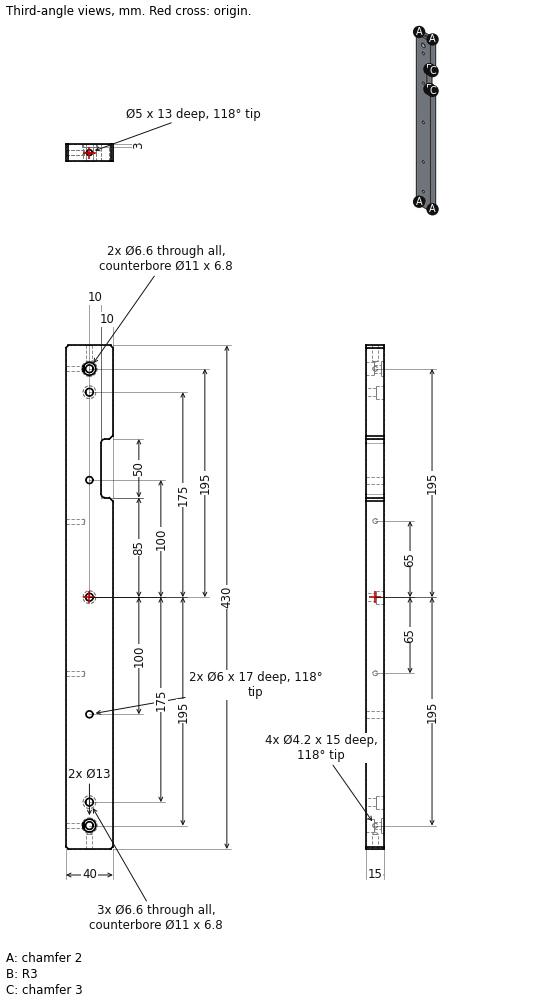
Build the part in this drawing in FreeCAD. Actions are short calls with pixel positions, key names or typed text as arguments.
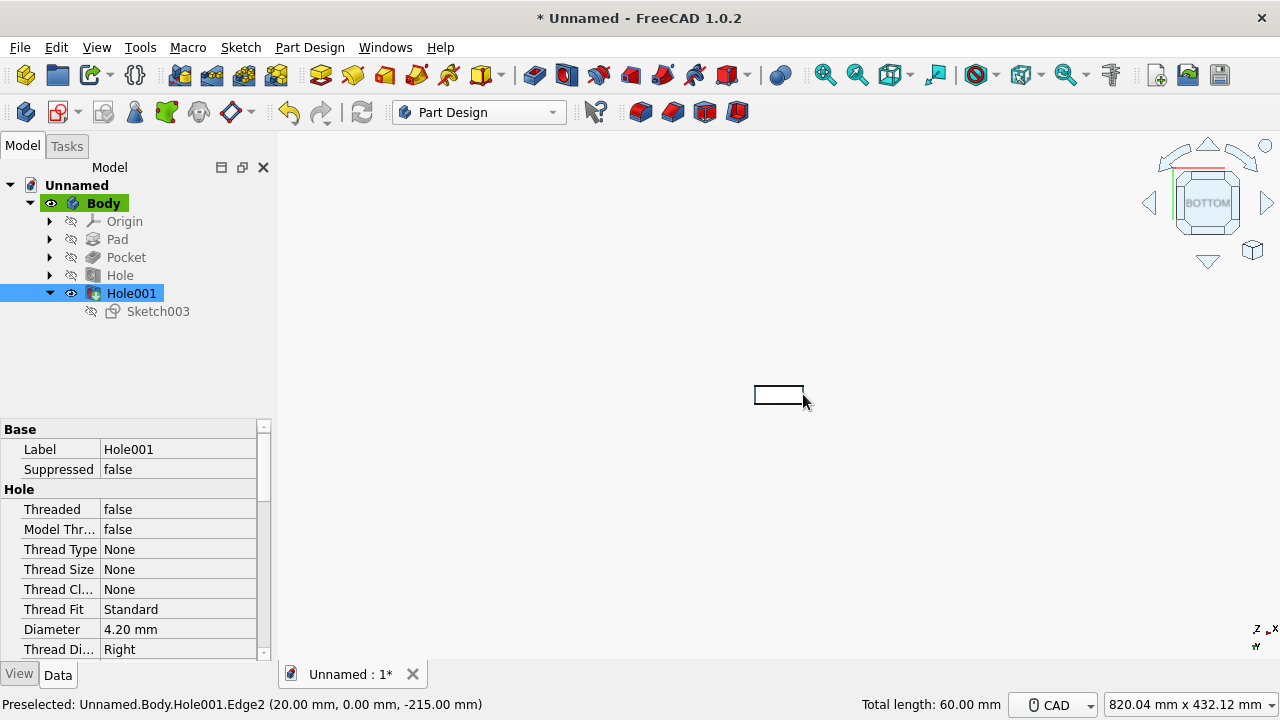
click(674, 112)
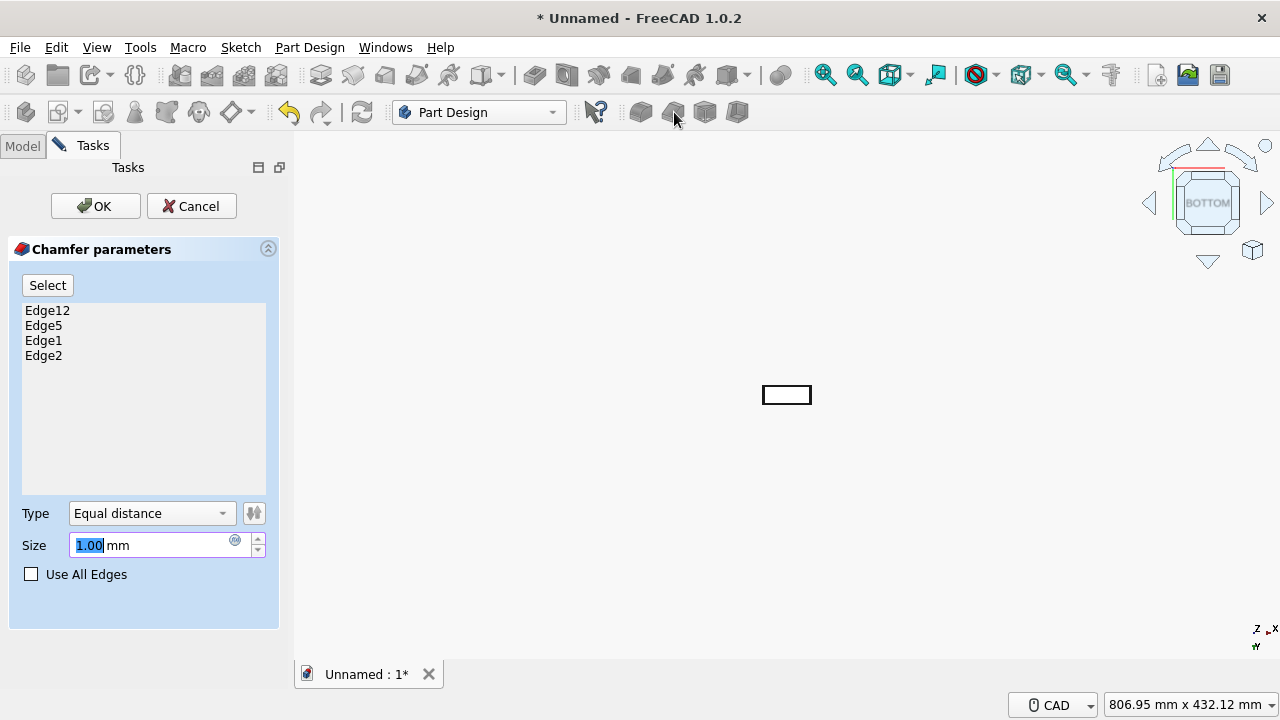
text(2)
key(Tab)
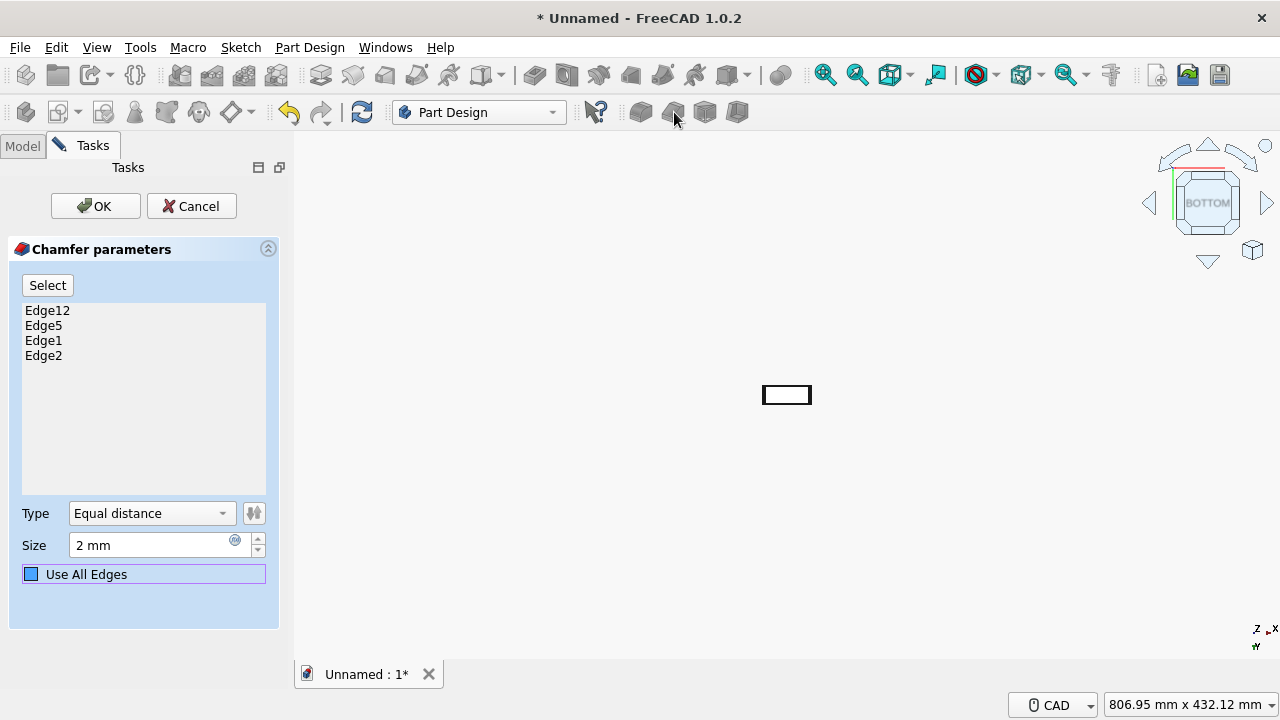
click(96, 206)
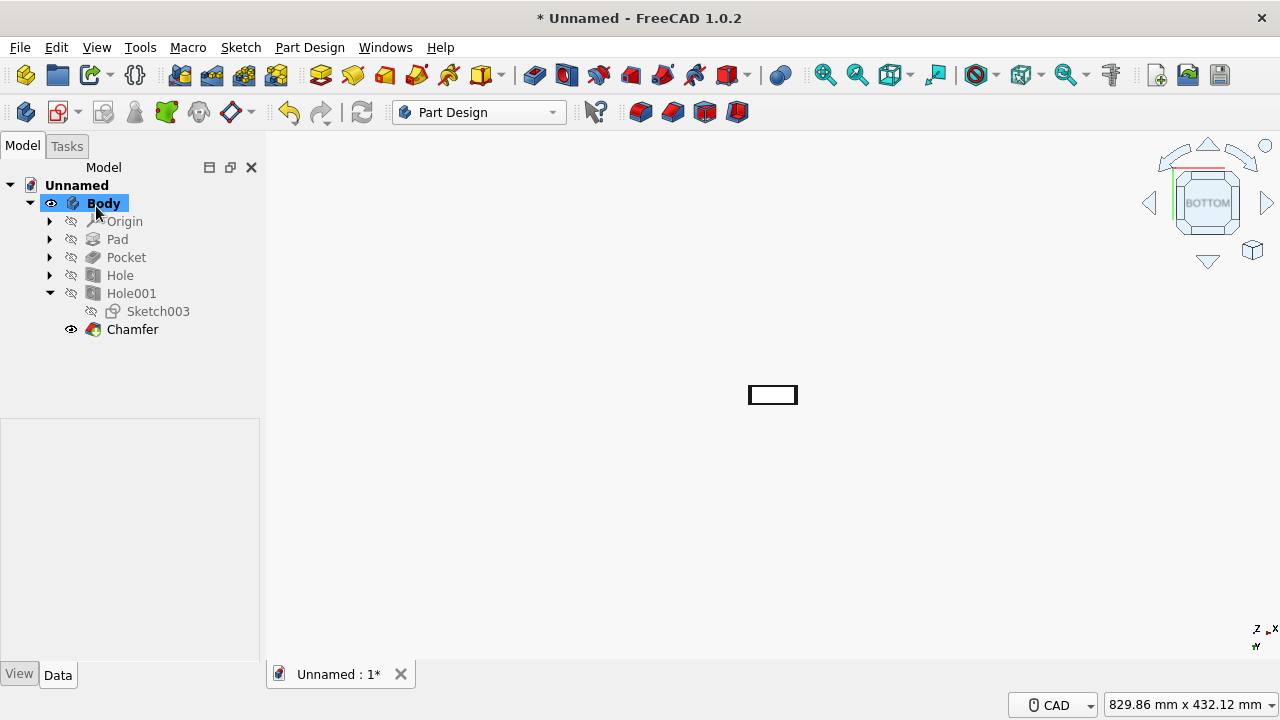
click(826, 76)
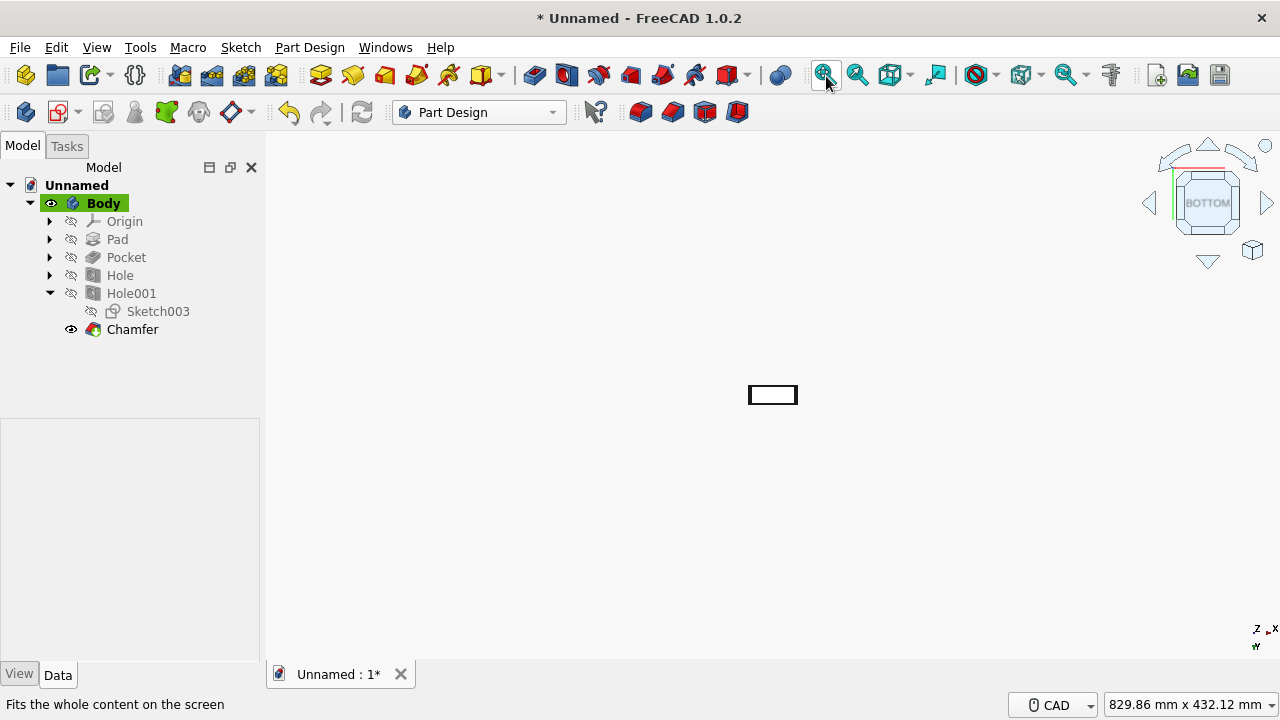
key(4)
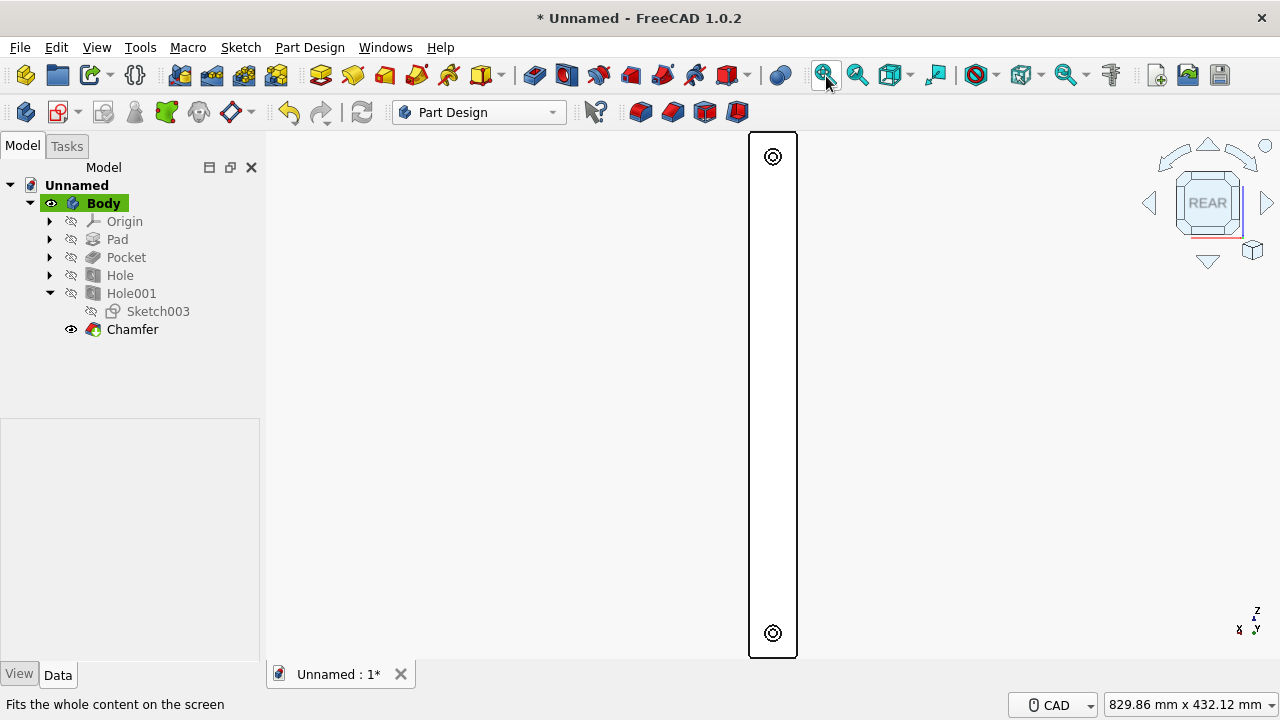
click(773, 244)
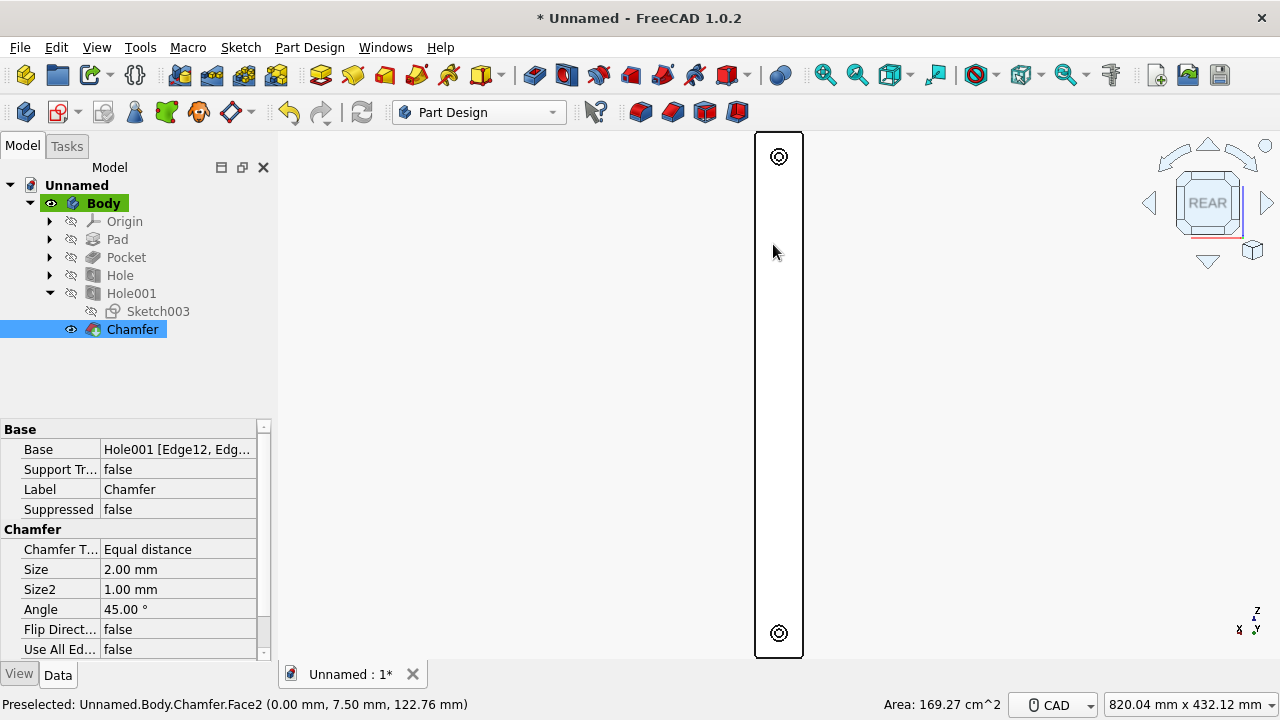
click(58, 112)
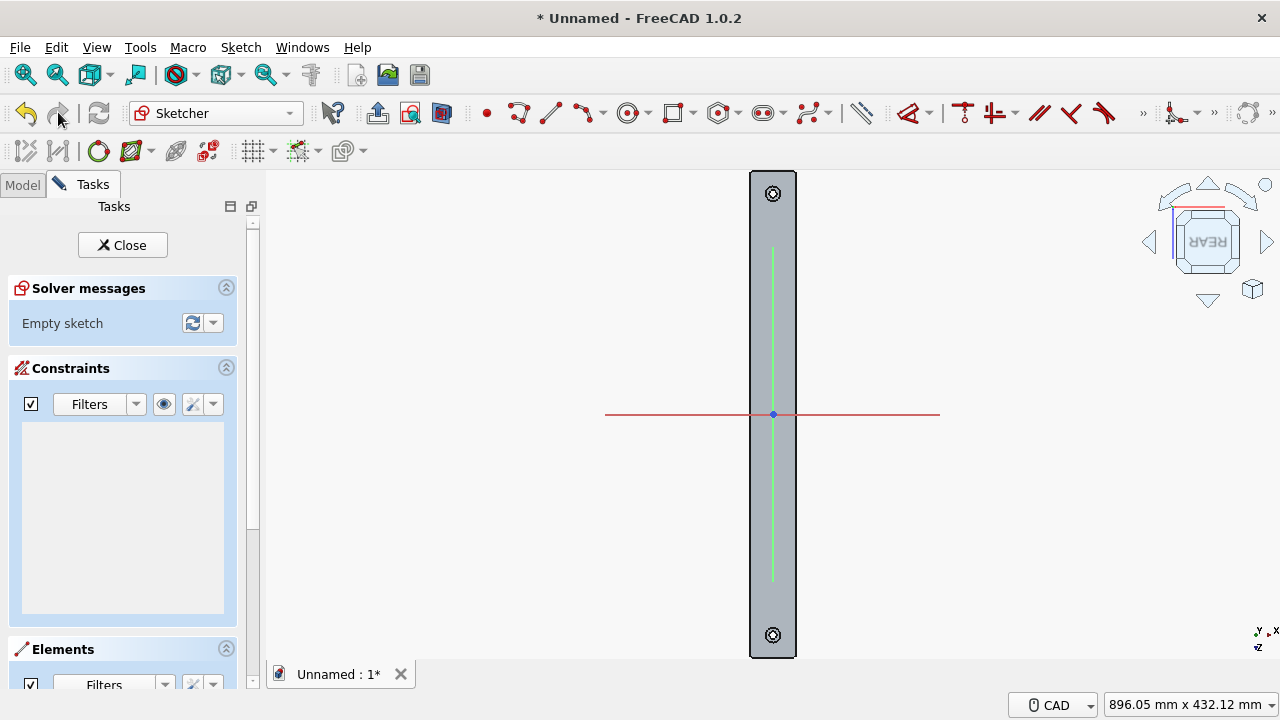
scroll(395, 414, down, 1)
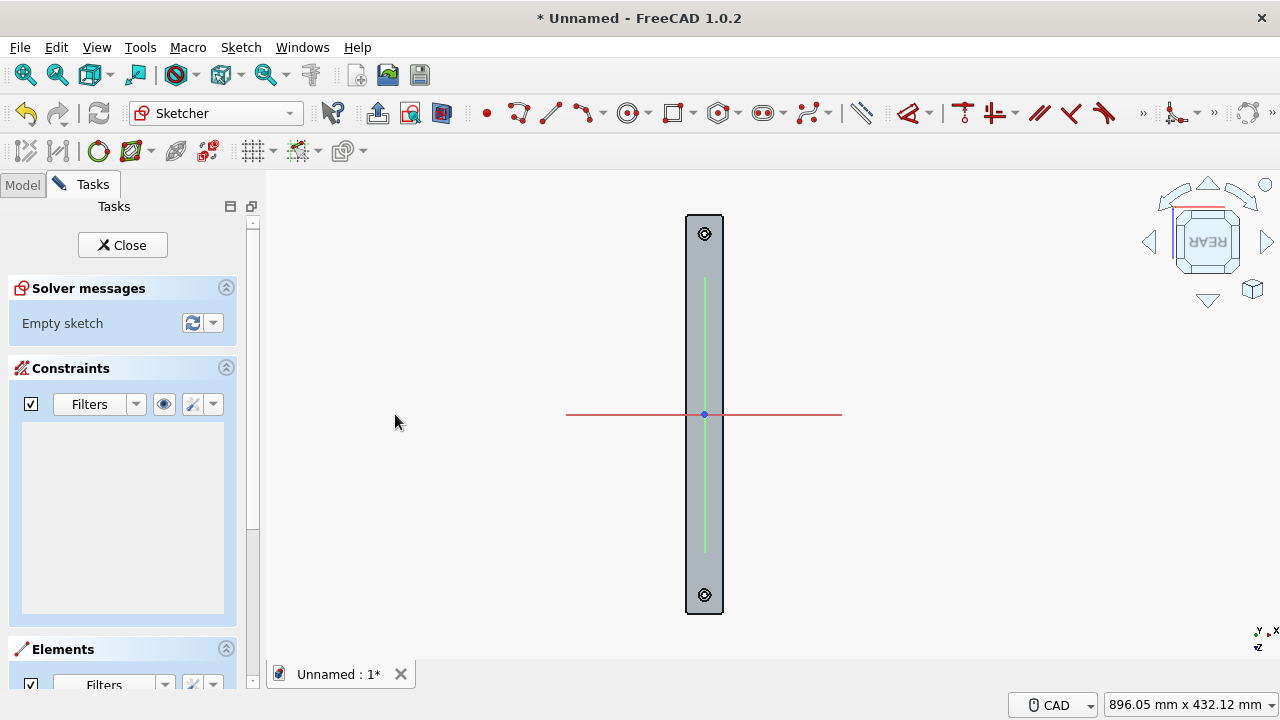
click(628, 114)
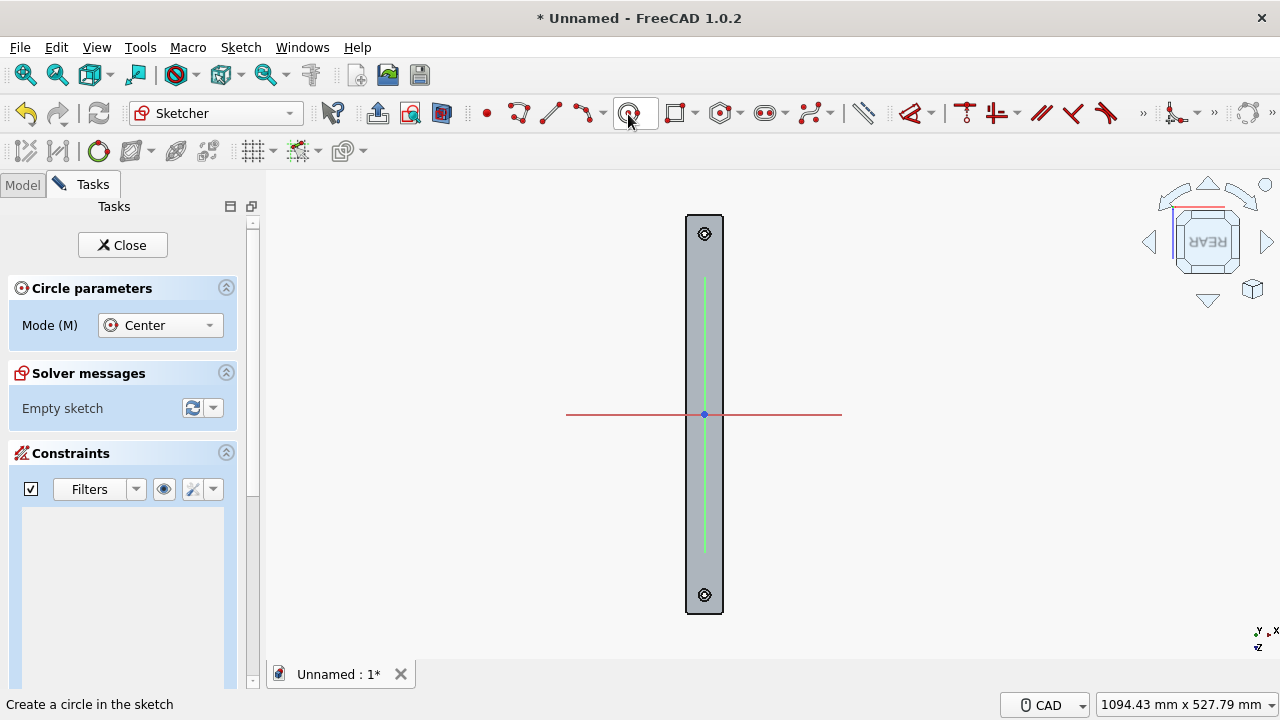
scroll(705, 252, up, 11)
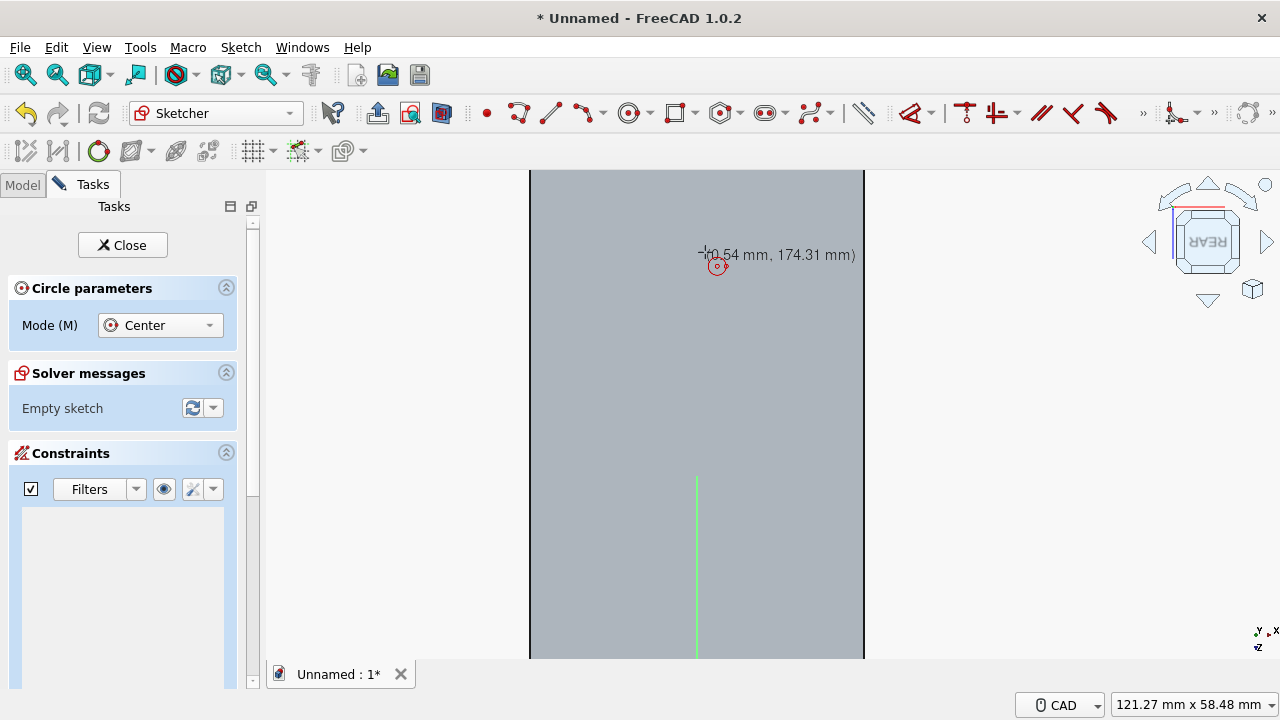
scroll(705, 252, down, 11)